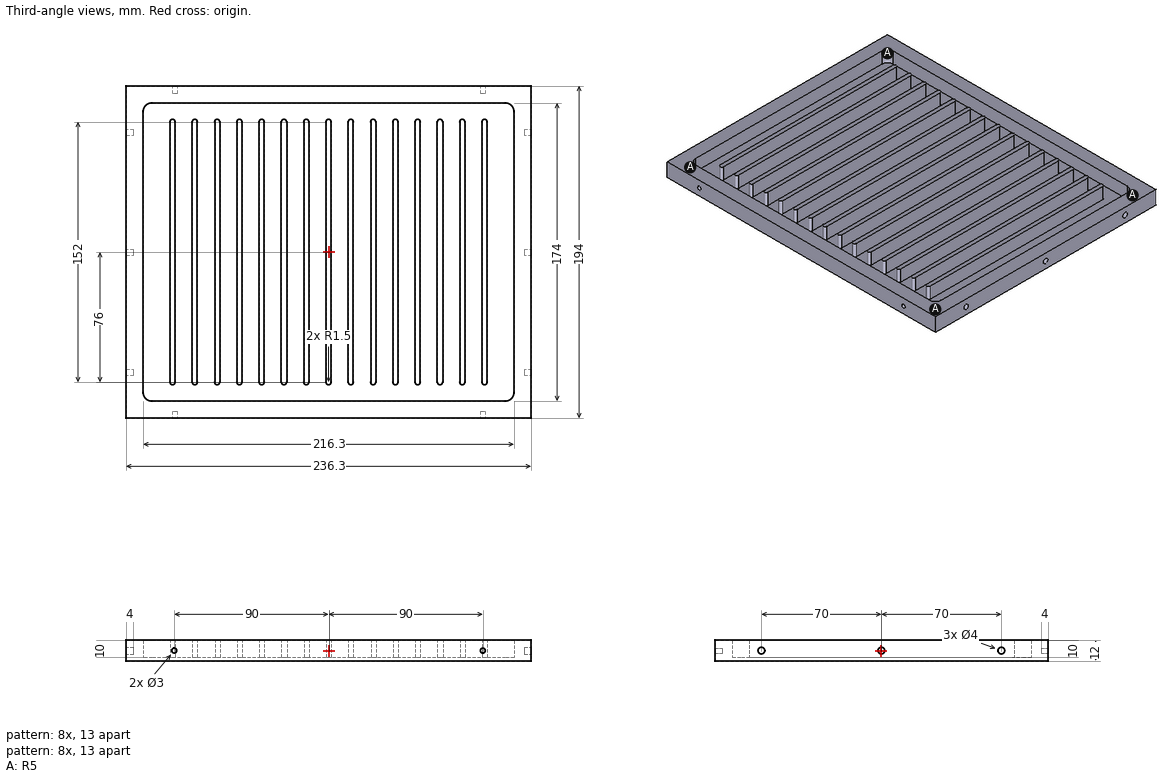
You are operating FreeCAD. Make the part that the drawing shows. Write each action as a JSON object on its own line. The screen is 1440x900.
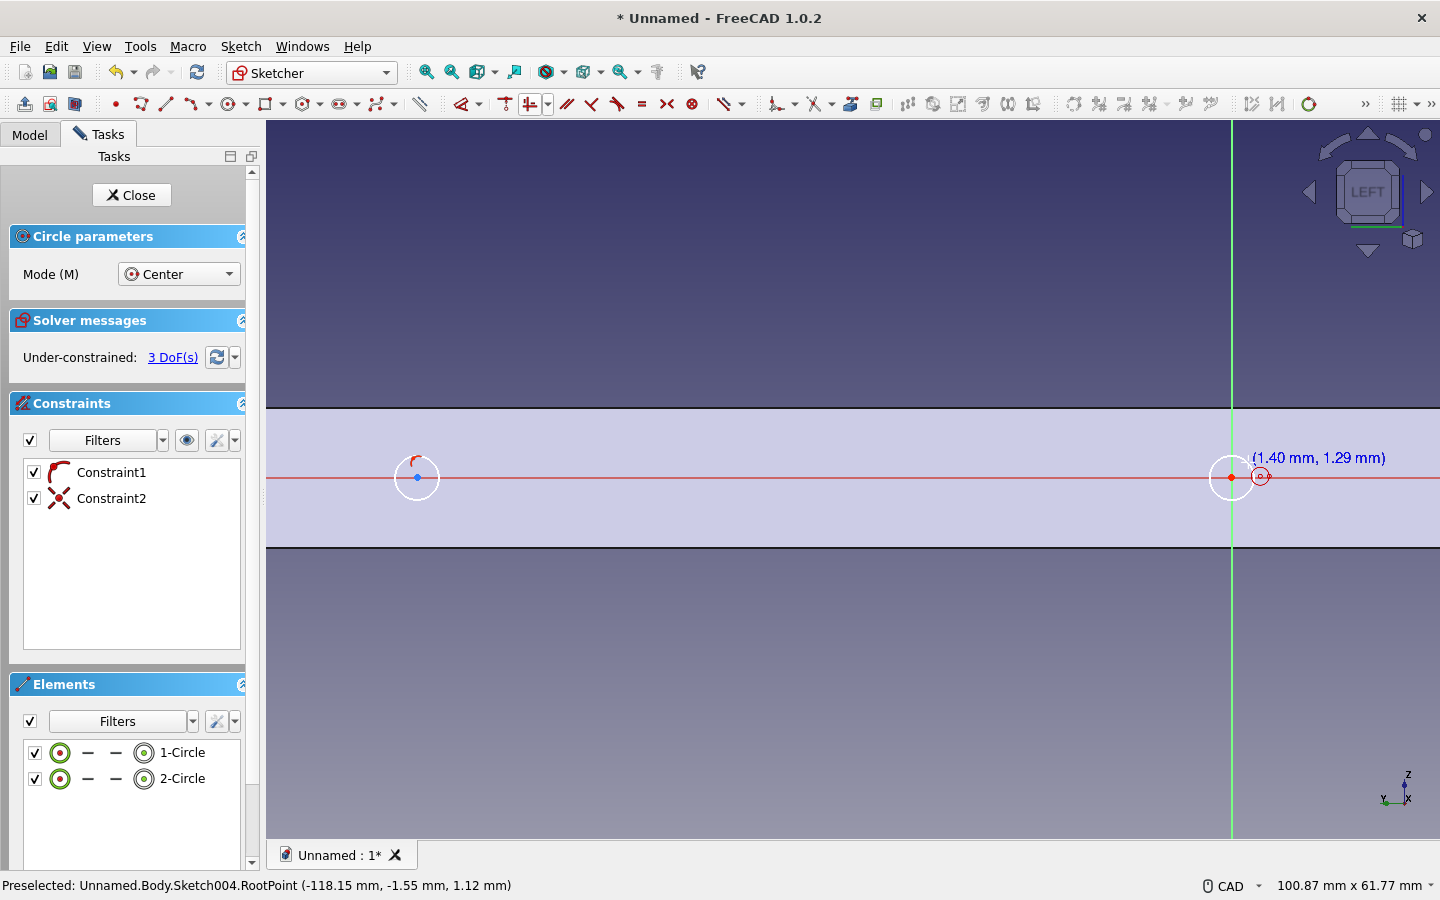
{"action": "scroll", "coordinate": [420, 481], "scroll_direction": "down", "scroll_amount": 4}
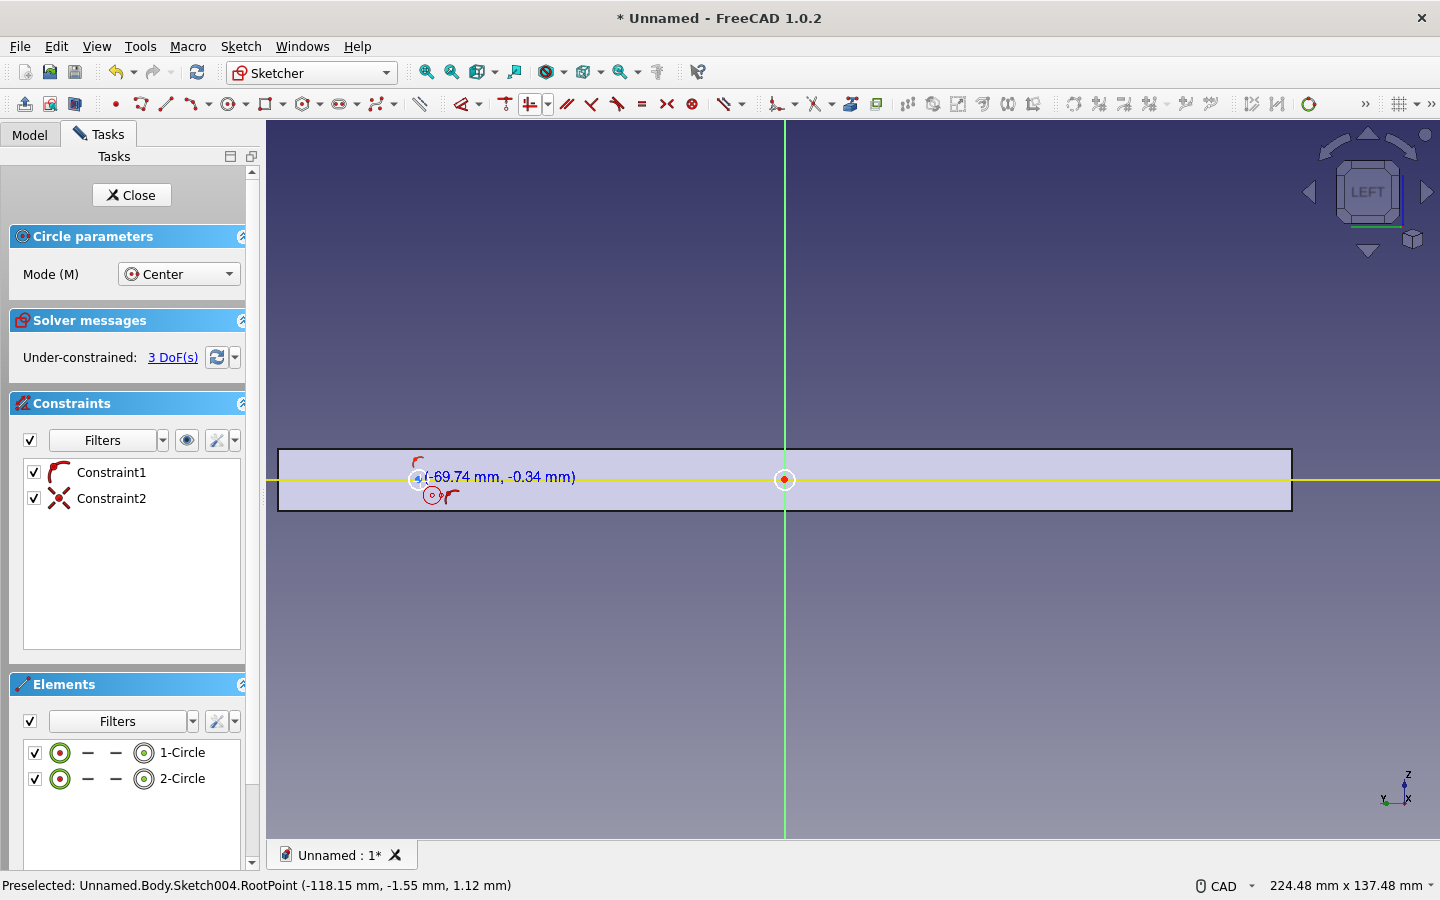
{"action": "scroll", "coordinate": [1151, 480], "scroll_direction": "up", "scroll_amount": 4}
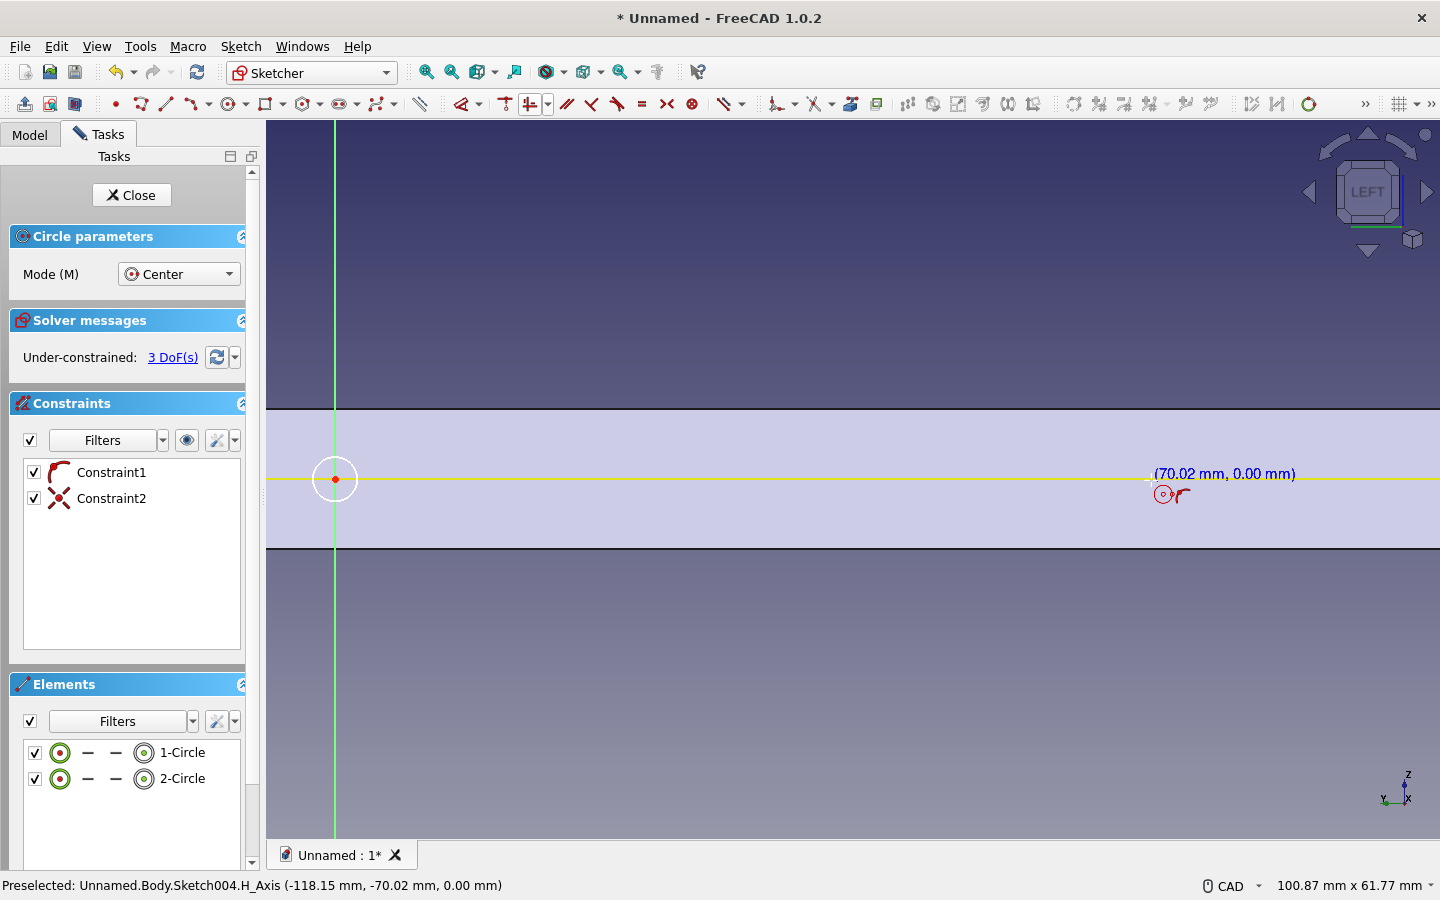
{"action": "left_click", "coordinate": [1150, 479]}
{"action": "left_click", "coordinate": [1166, 463]}
{"action": "key", "text": "Escape"}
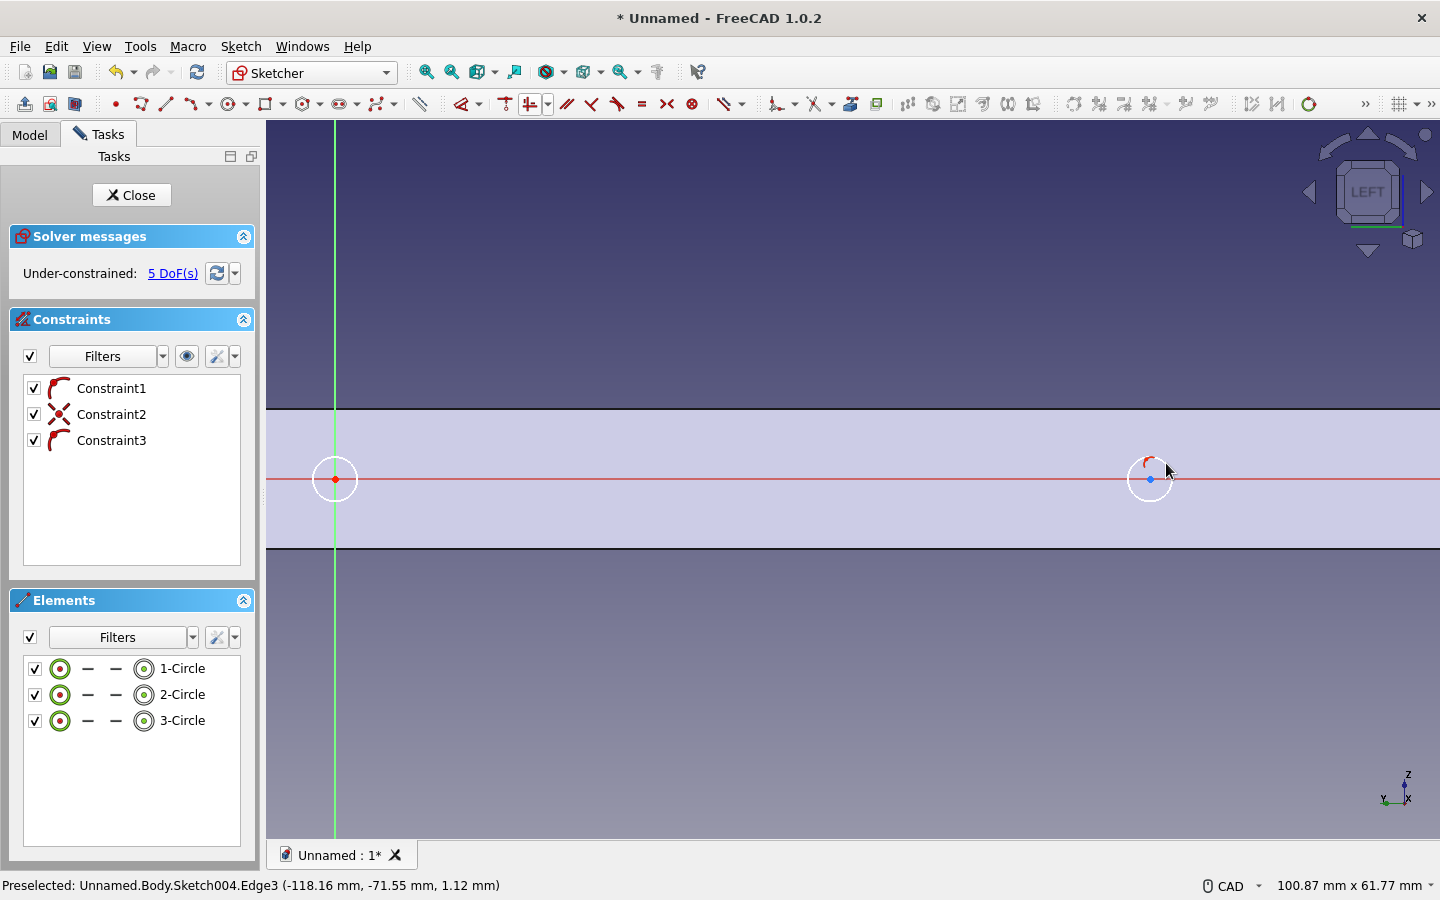
{"action": "scroll", "coordinate": [1151, 480], "scroll_direction": "down", "scroll_amount": 4}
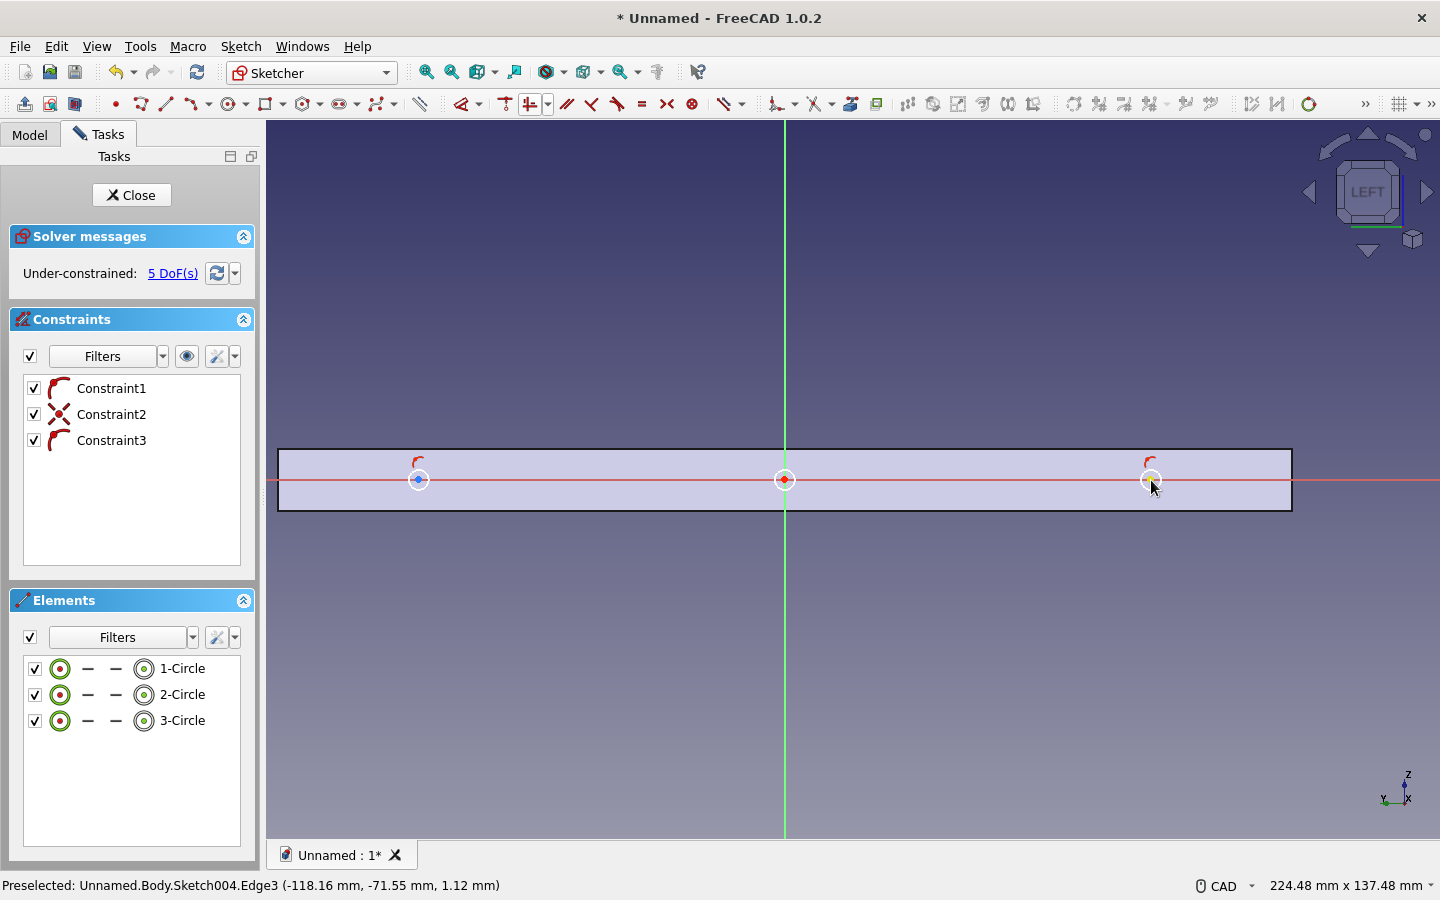
{"action": "scroll", "coordinate": [426, 473], "scroll_direction": "up", "scroll_amount": 4}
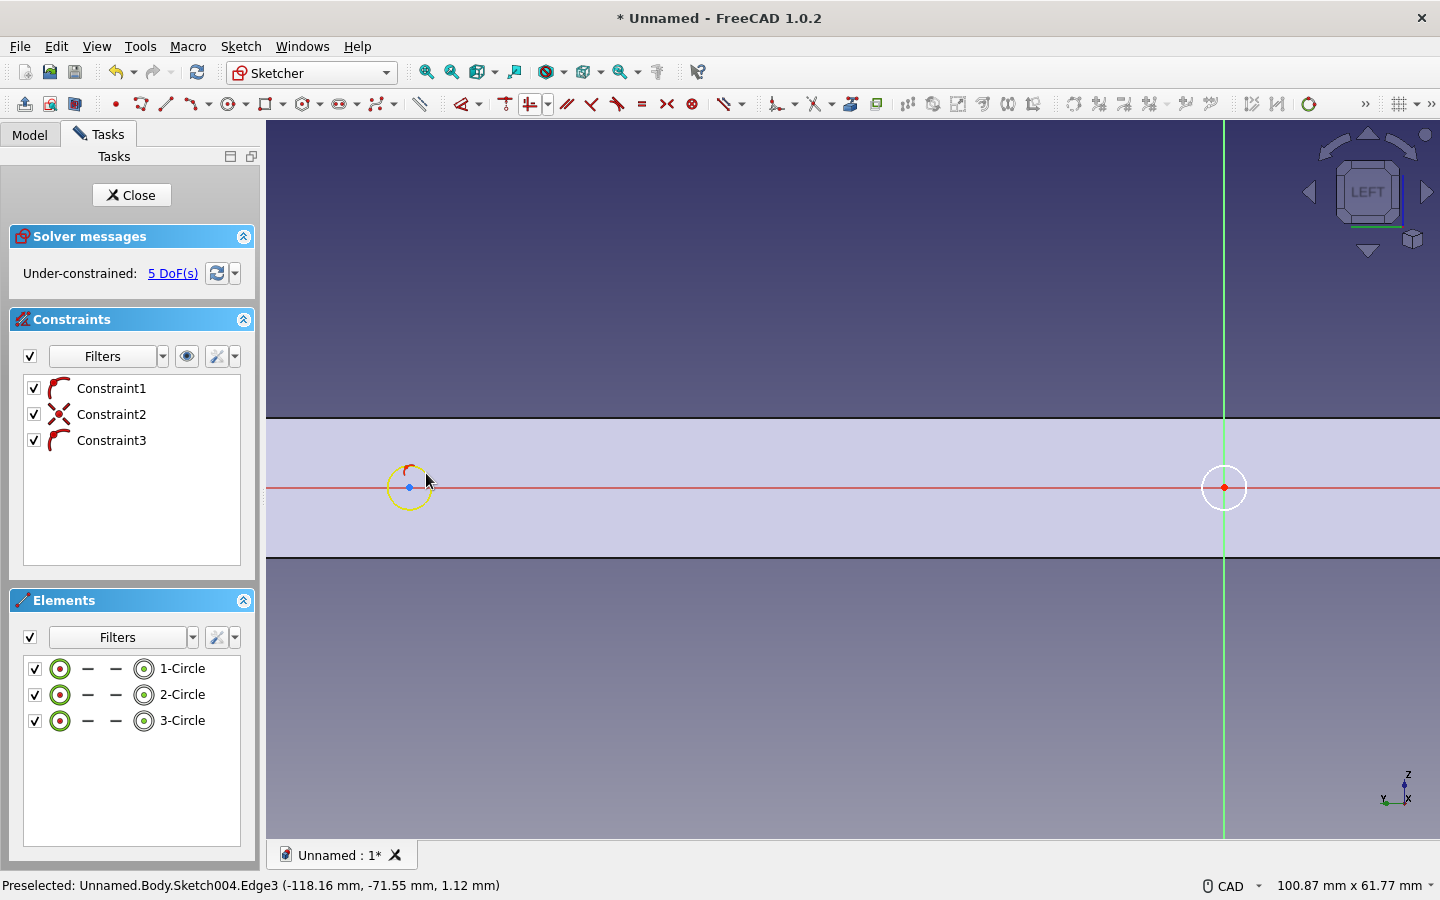
{"action": "left_click", "coordinate": [425, 472]}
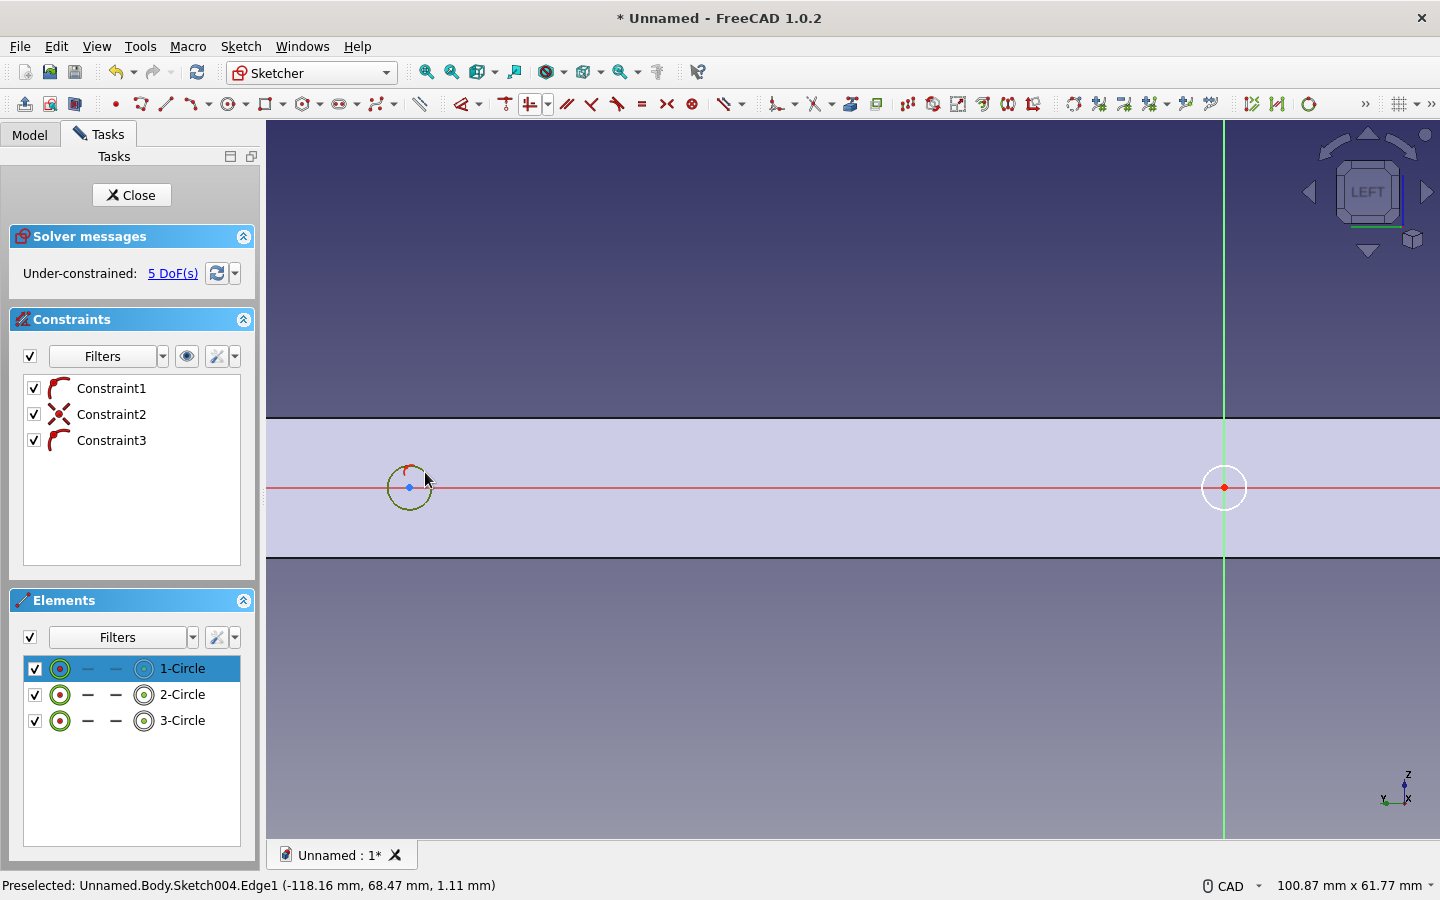
{"action": "left_click", "coordinate": [1240, 472]}